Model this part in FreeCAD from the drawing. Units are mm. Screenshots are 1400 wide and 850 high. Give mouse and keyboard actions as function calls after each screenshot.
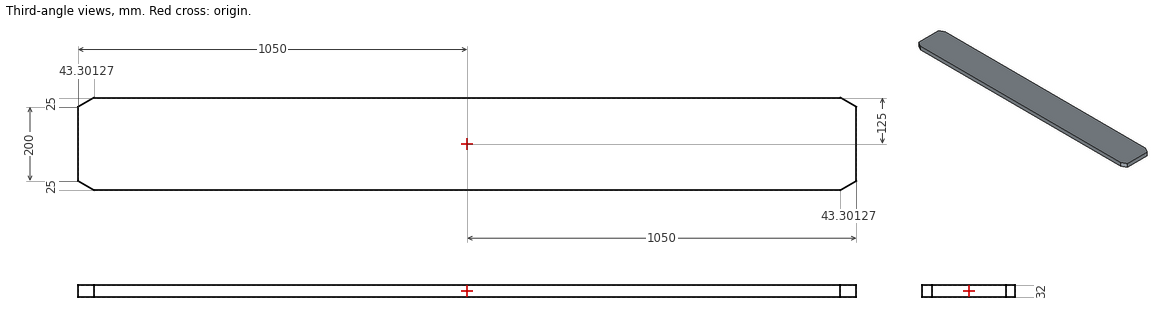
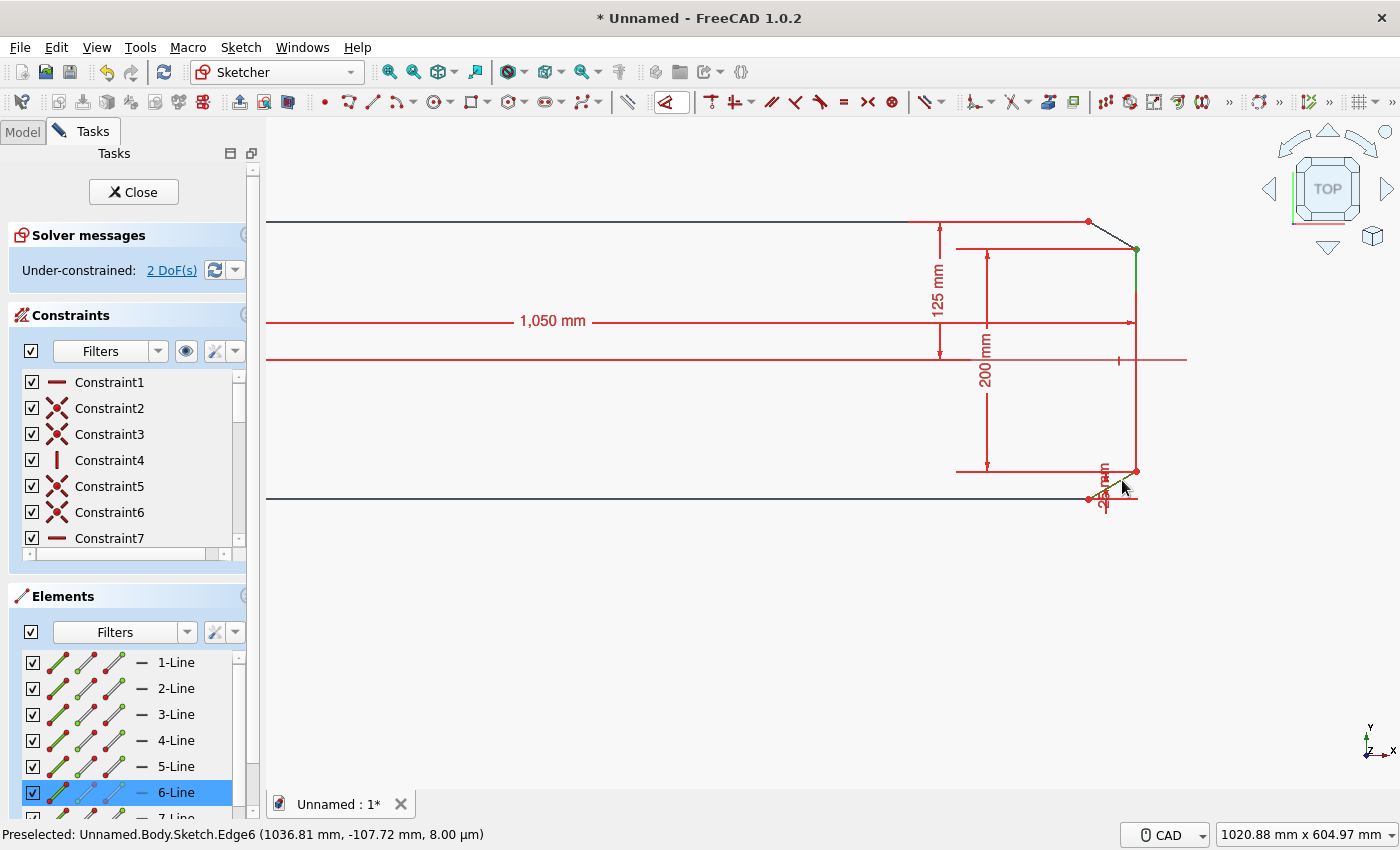
click(684, 102)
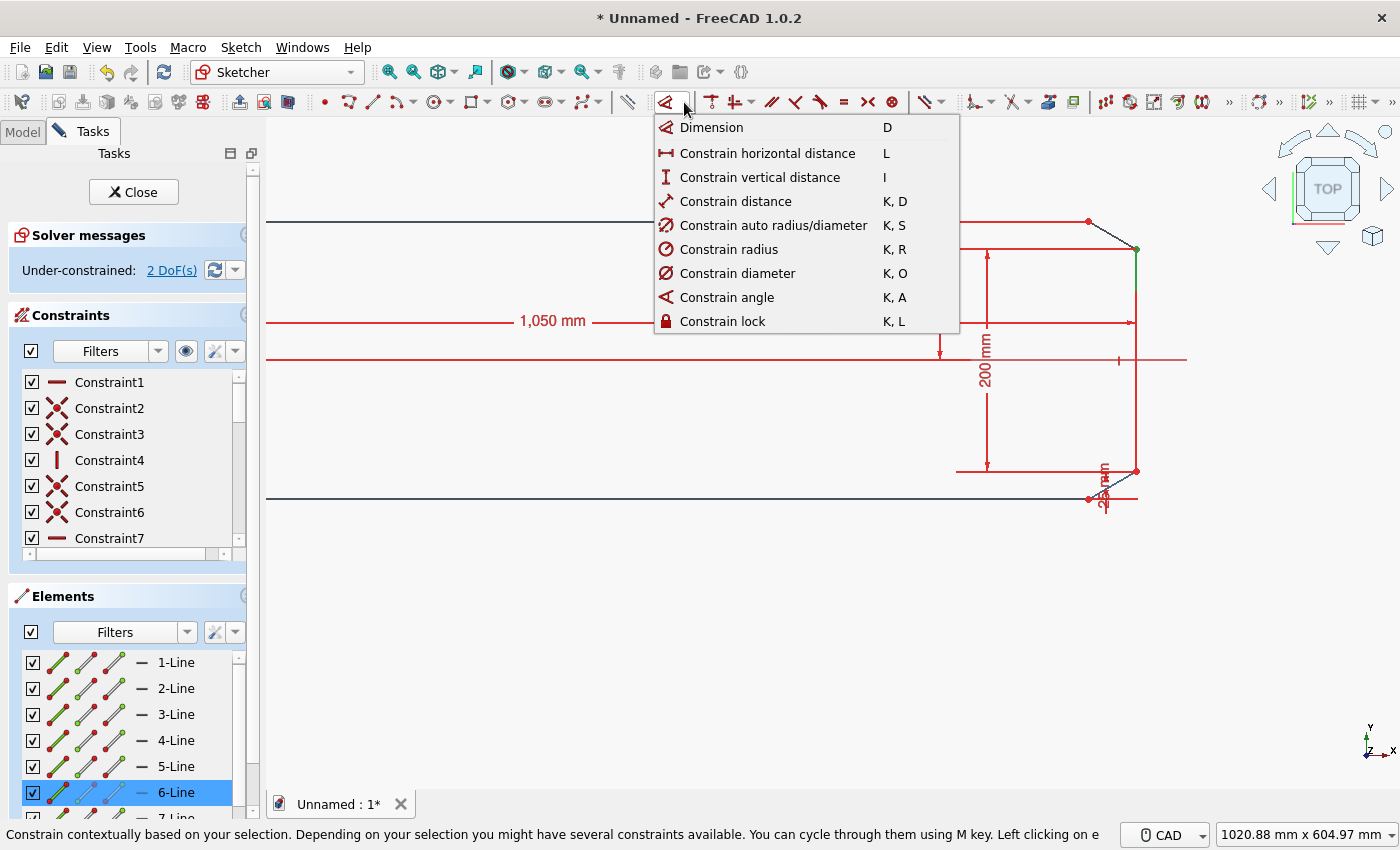
click(807, 153)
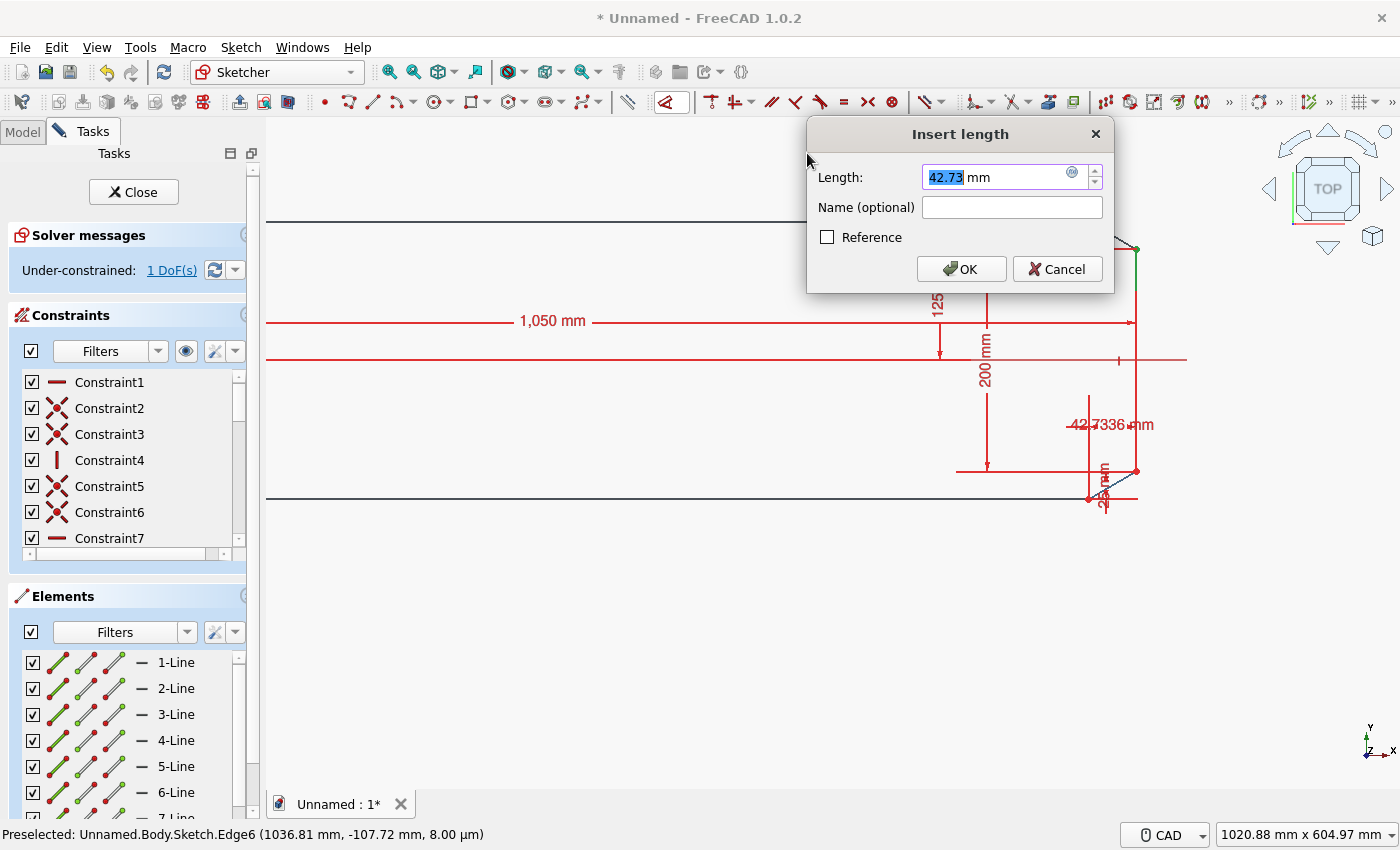
text(43.30127)
key(Return)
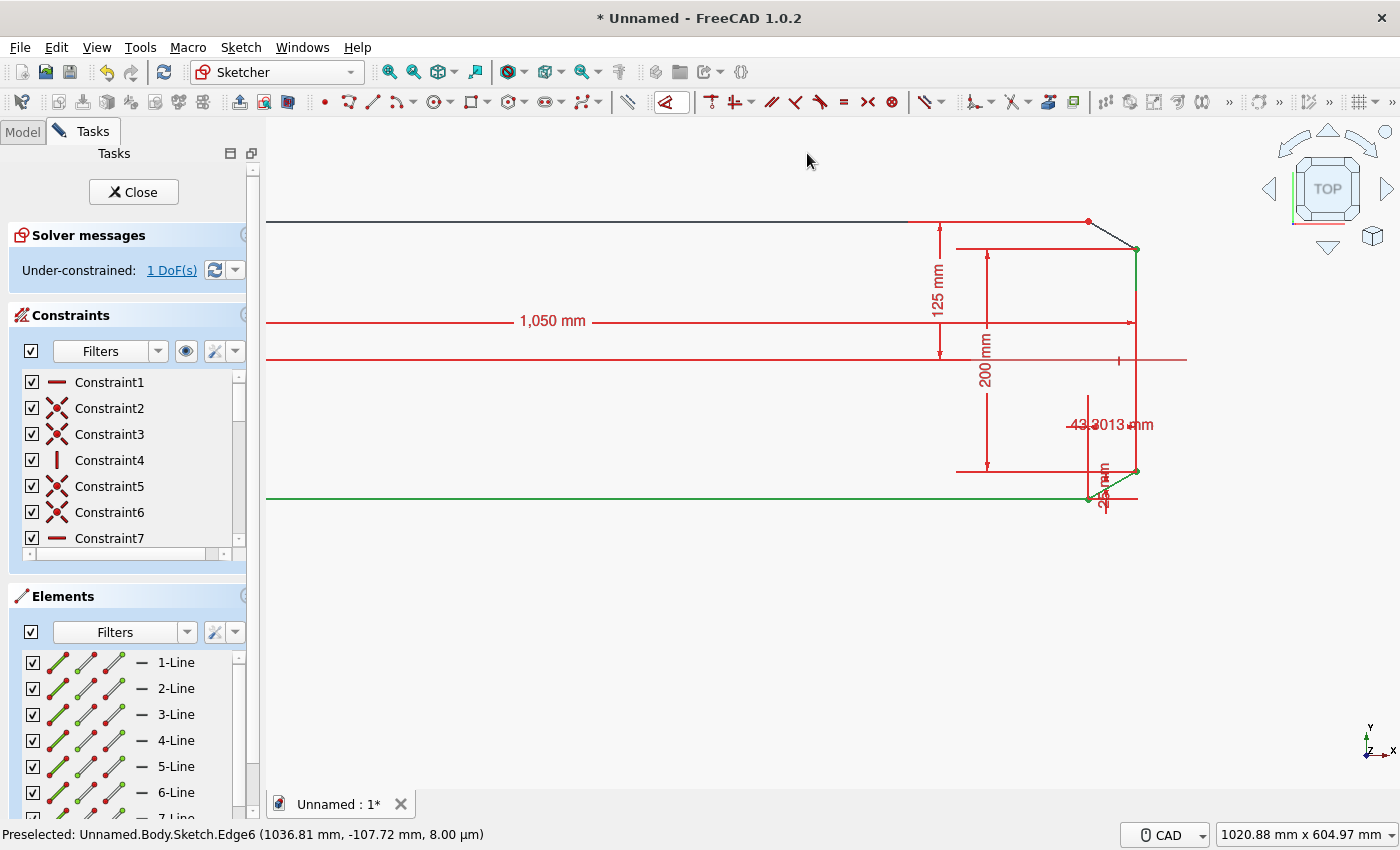
click(1122, 241)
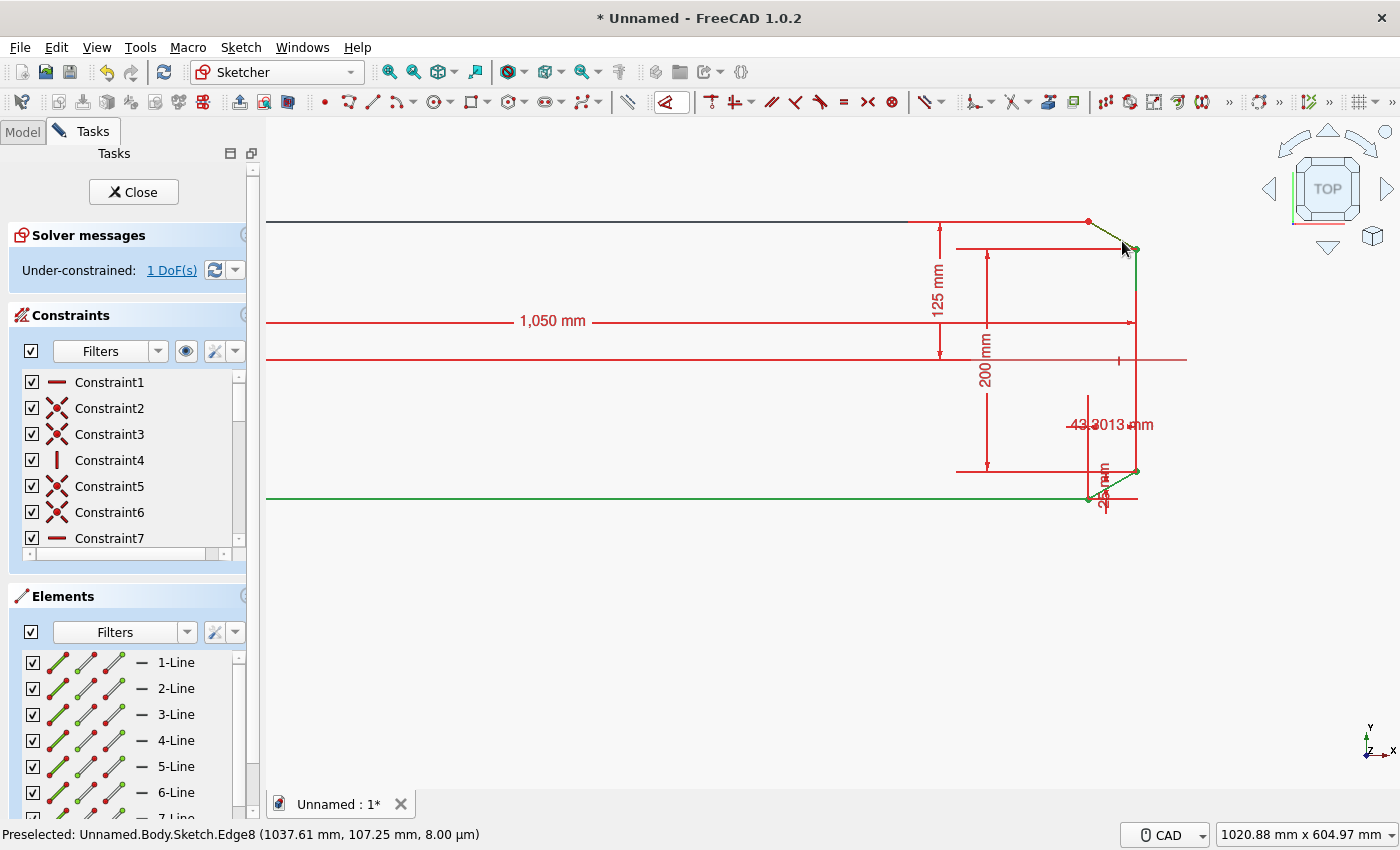
click(684, 102)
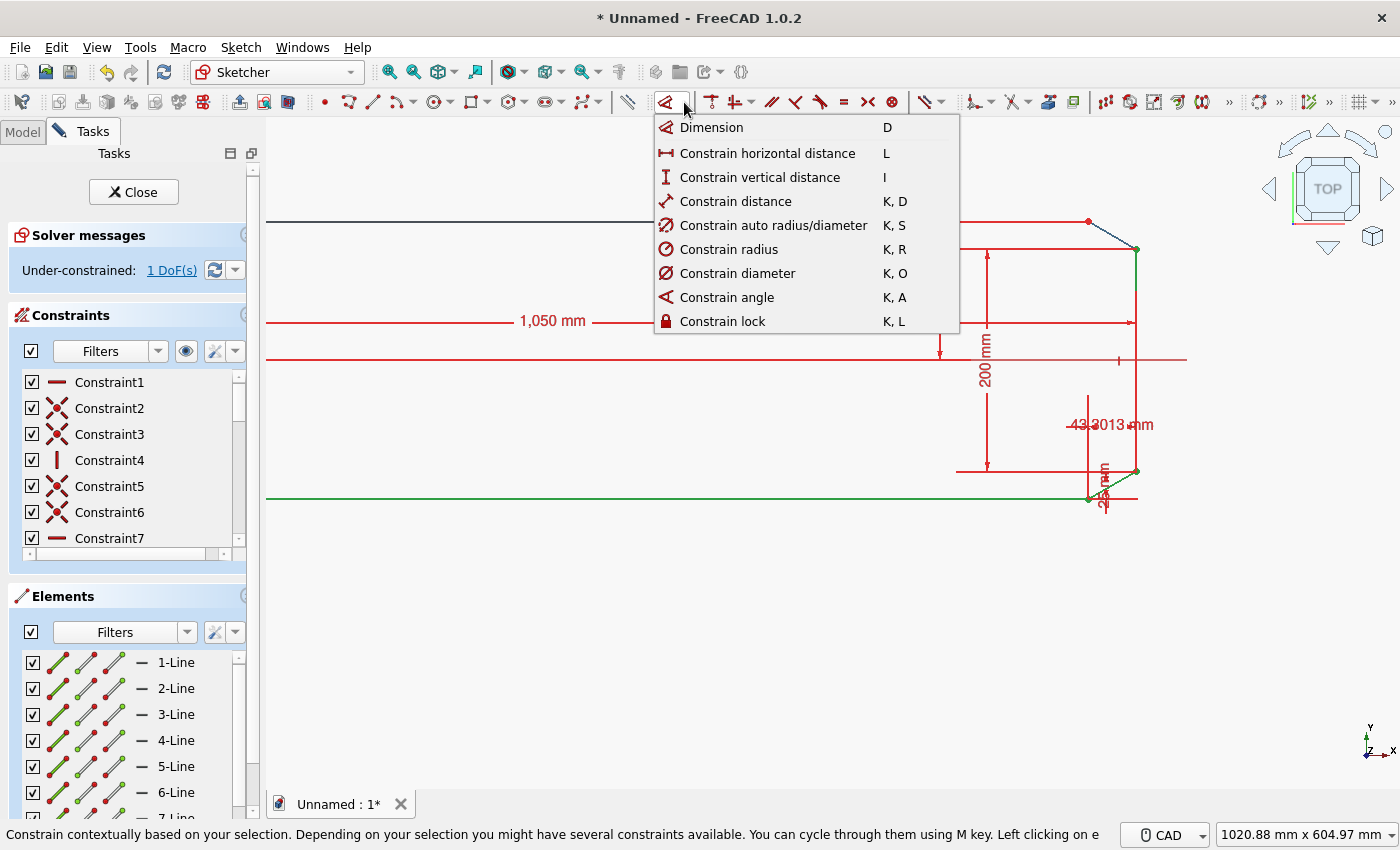
click(807, 153)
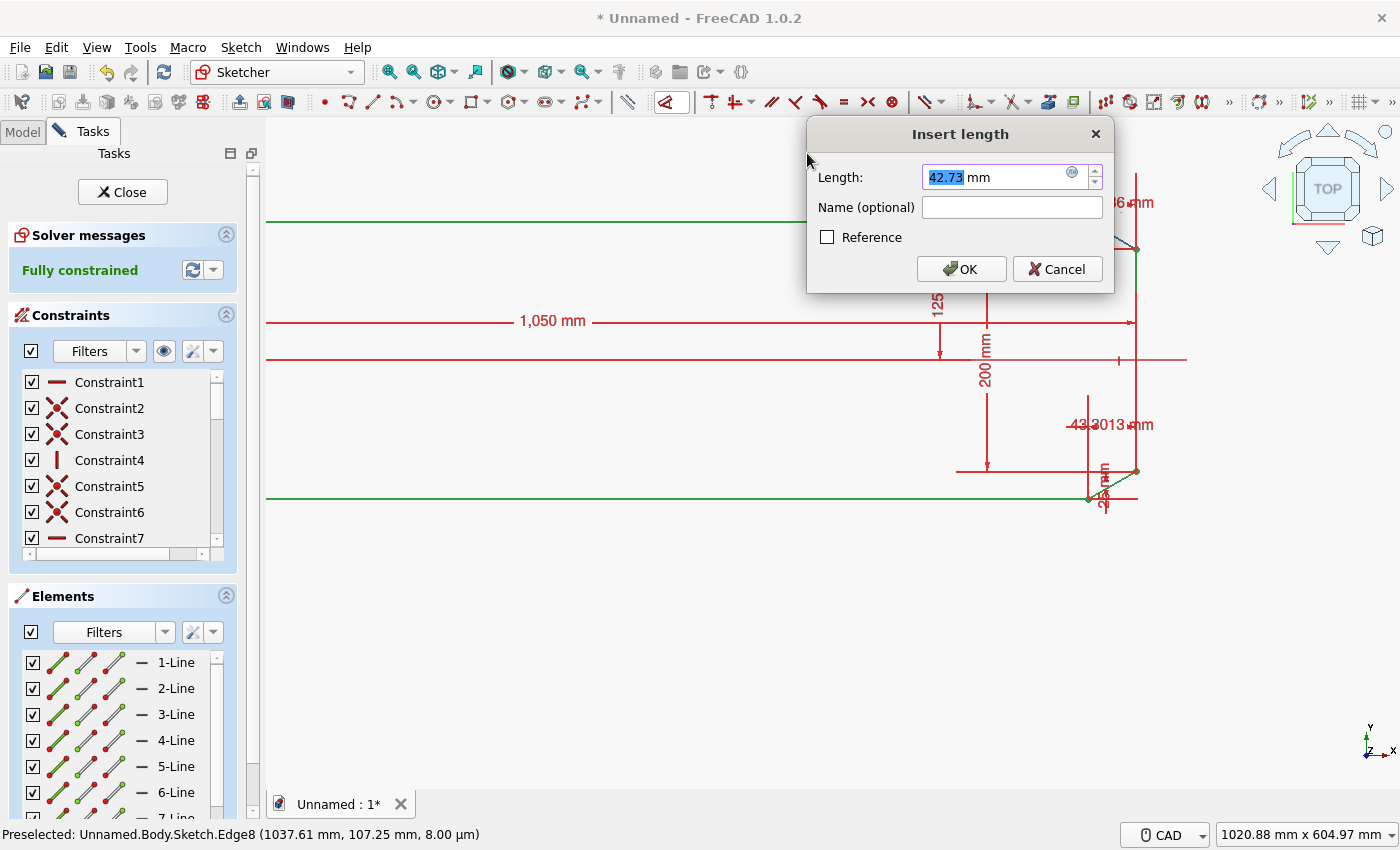
text(43.30127)
key(Return)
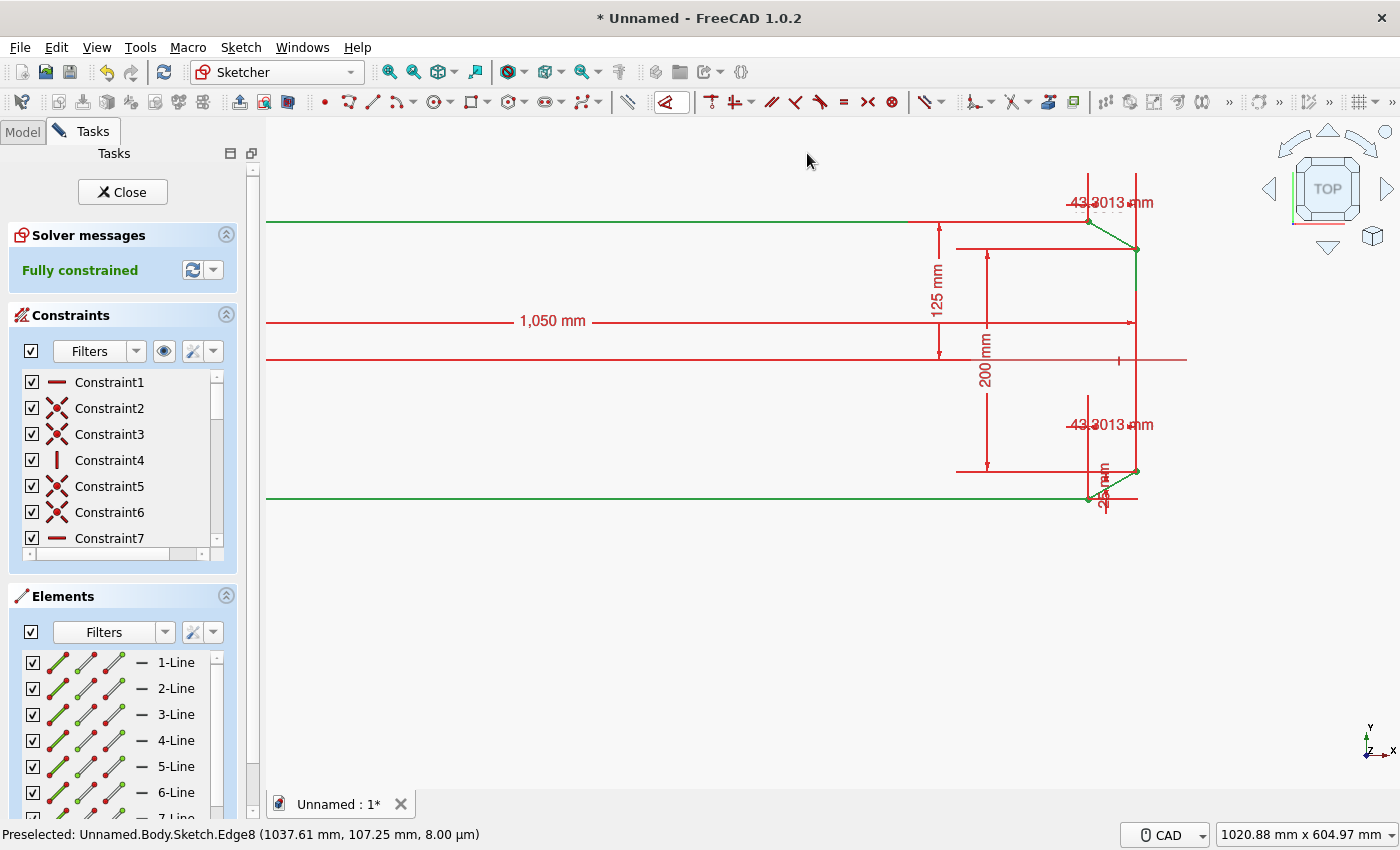
click(123, 192)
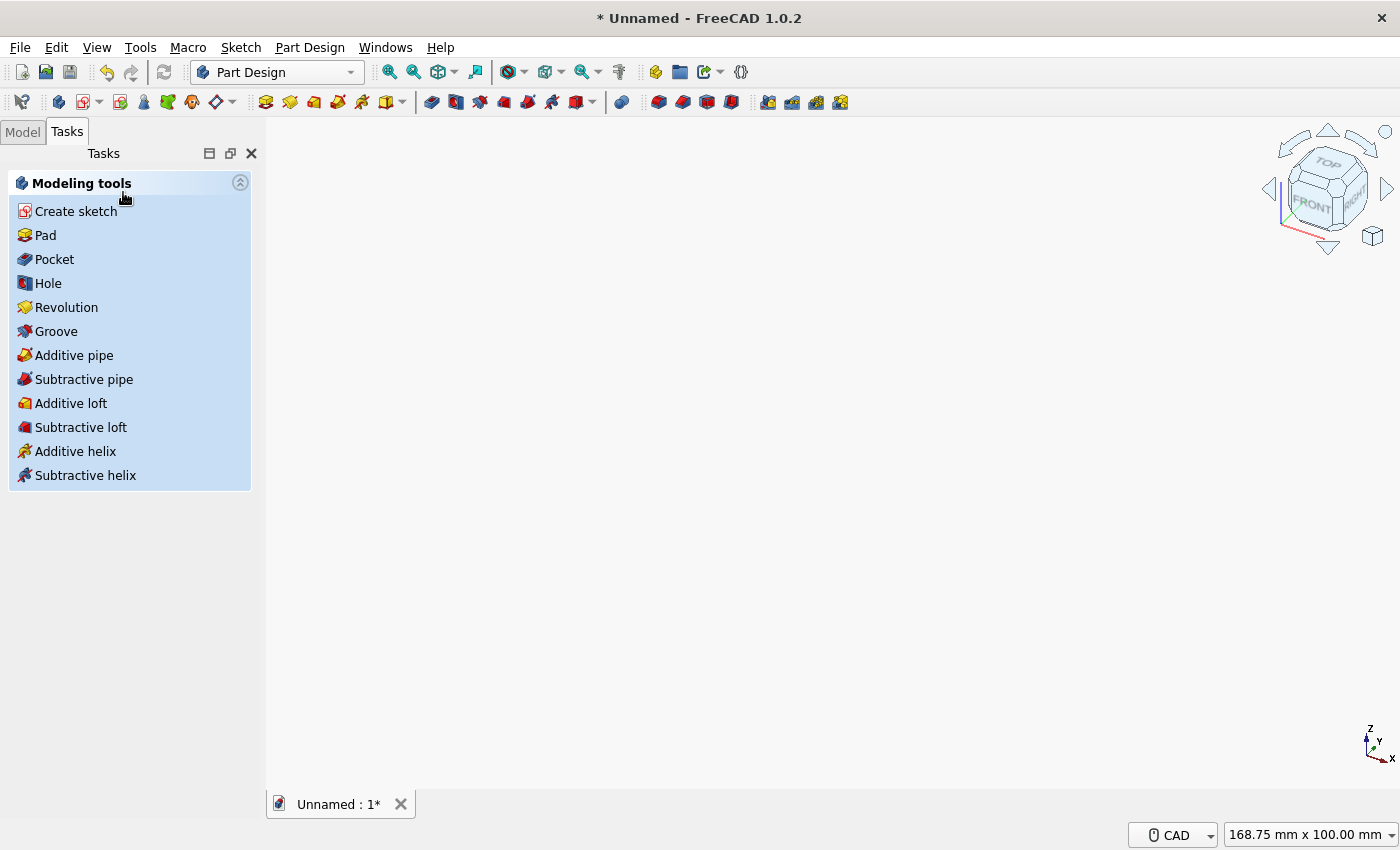
click(266, 102)